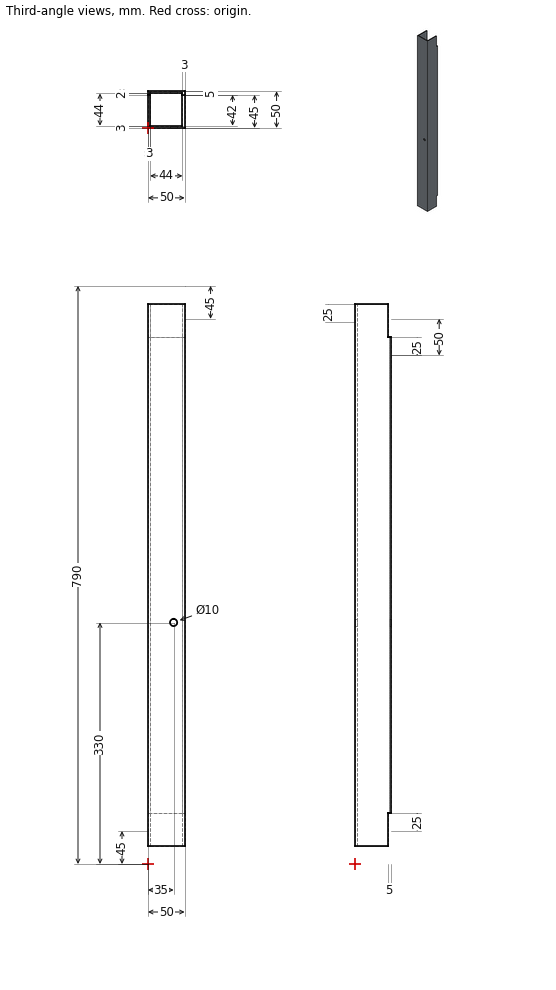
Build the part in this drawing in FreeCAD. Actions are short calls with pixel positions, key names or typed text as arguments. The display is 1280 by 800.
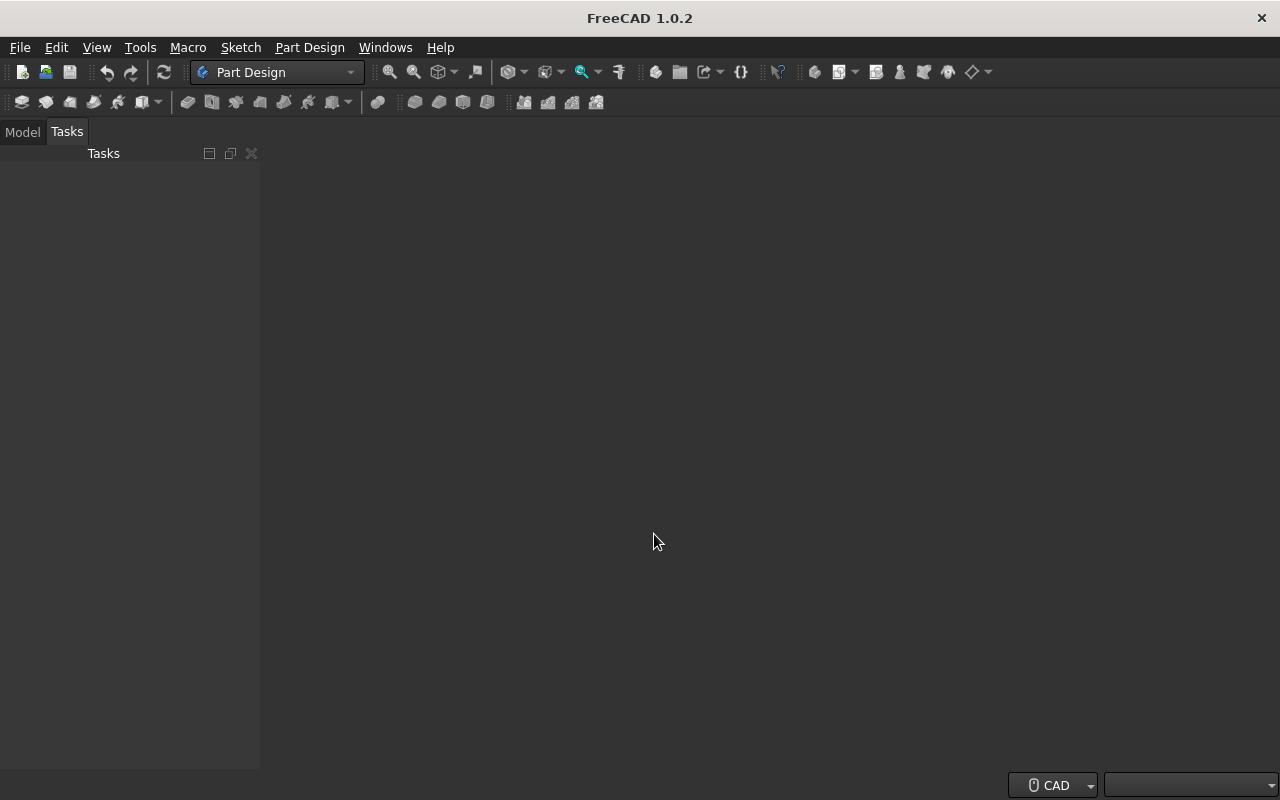
click(22, 72)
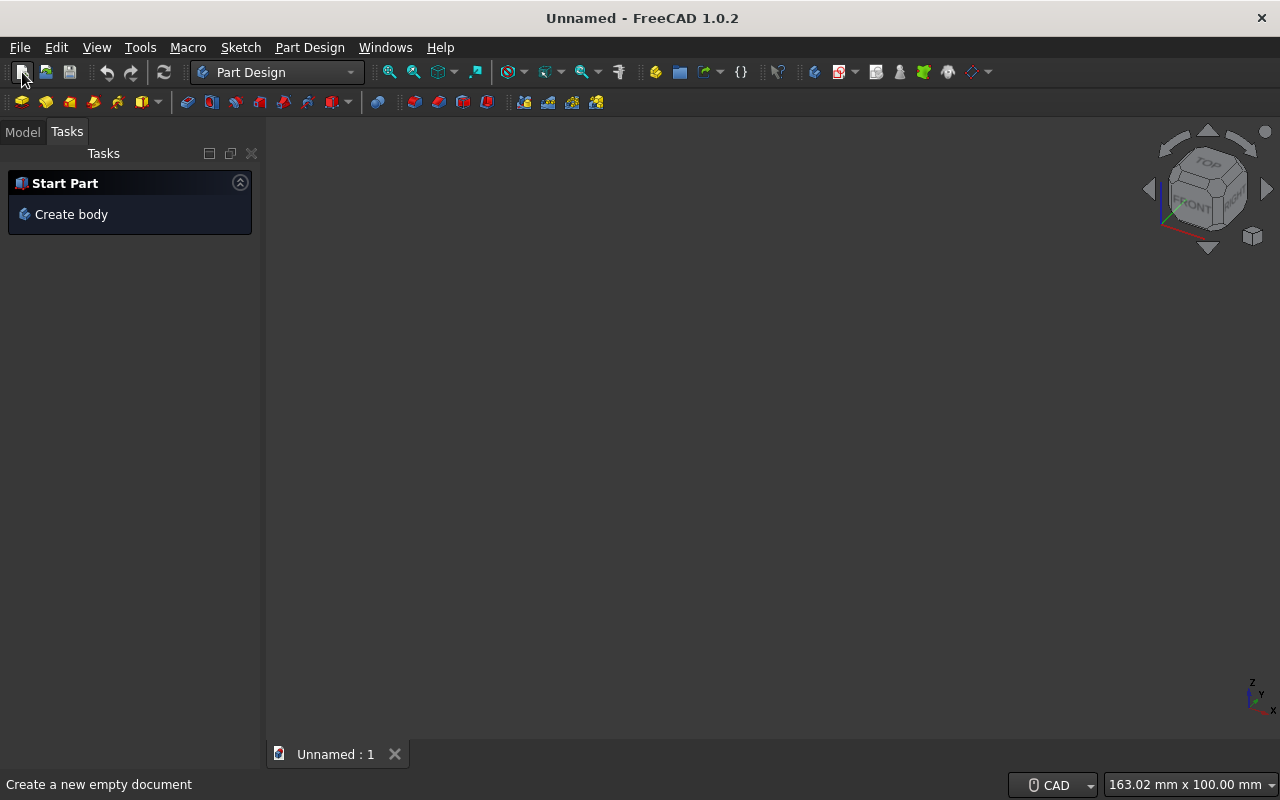
click(840, 72)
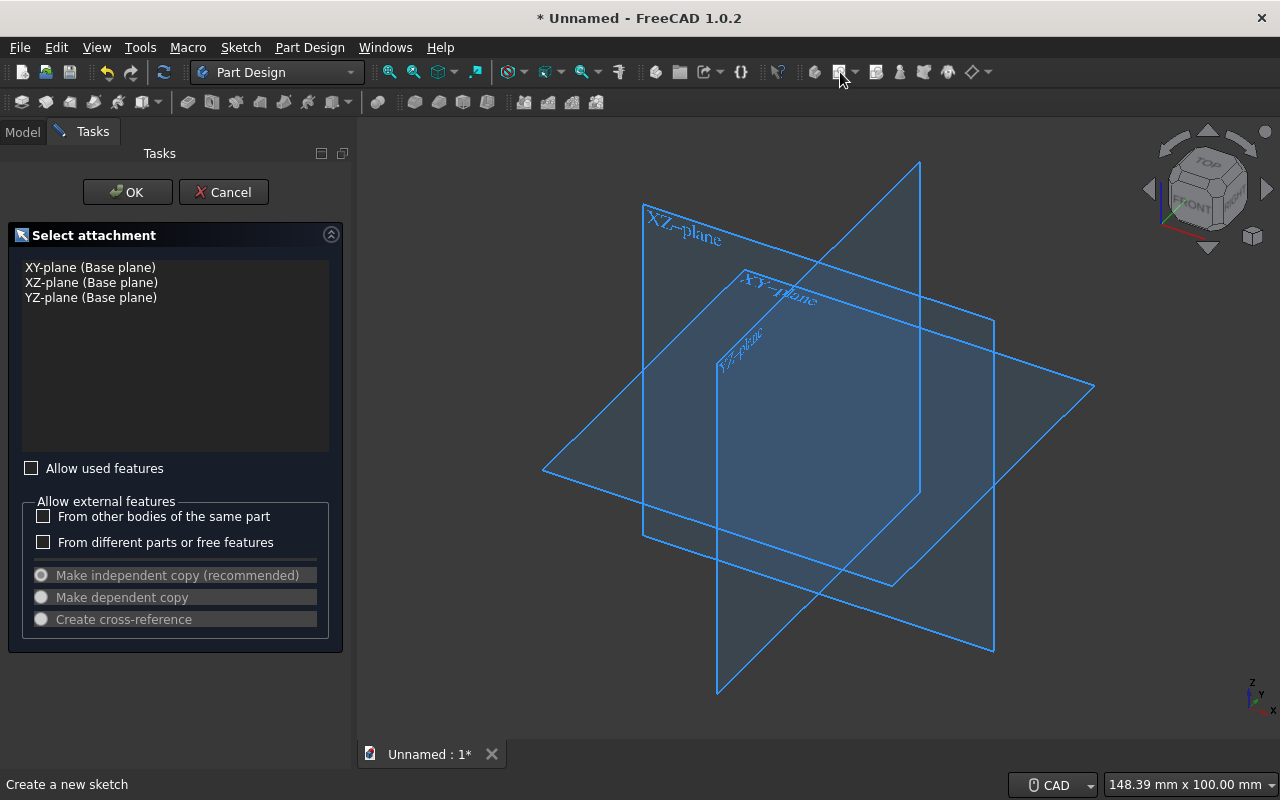
click(82, 268)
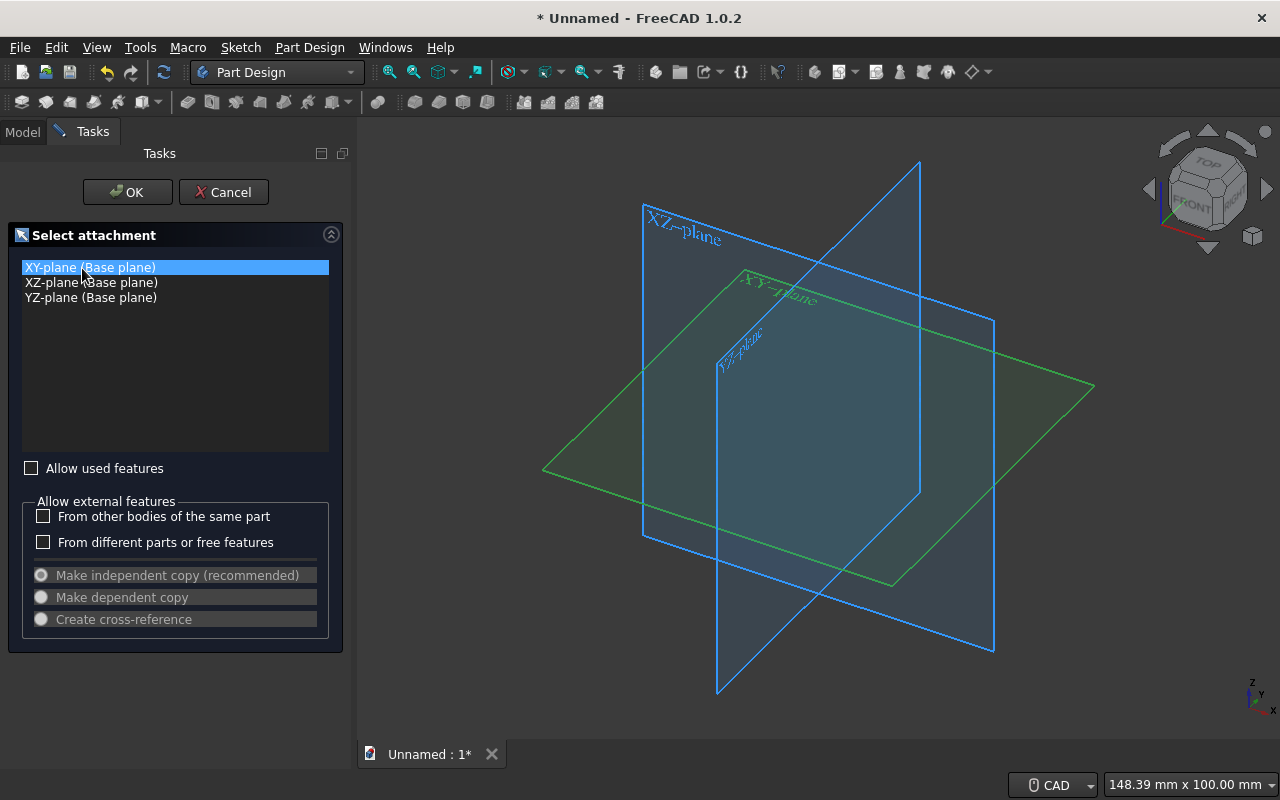
click(128, 192)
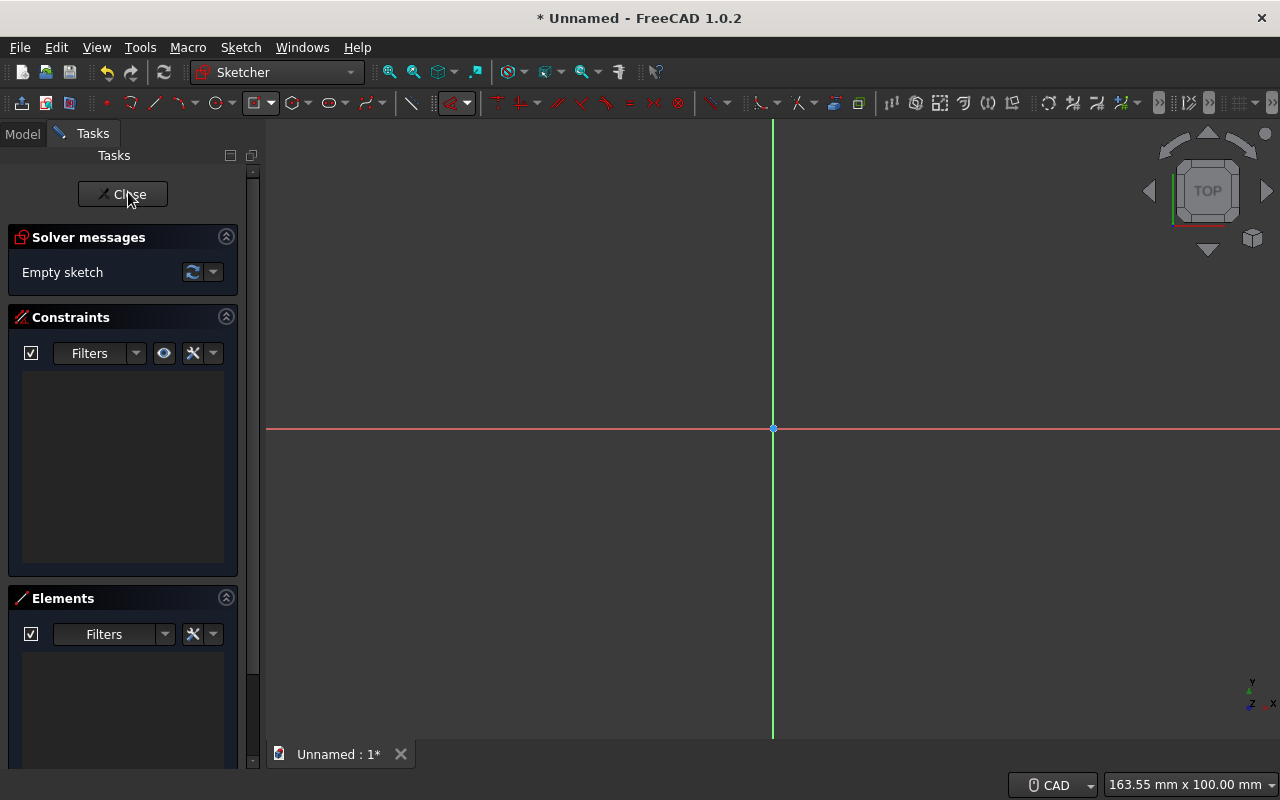
scroll(294, 711, down, 1)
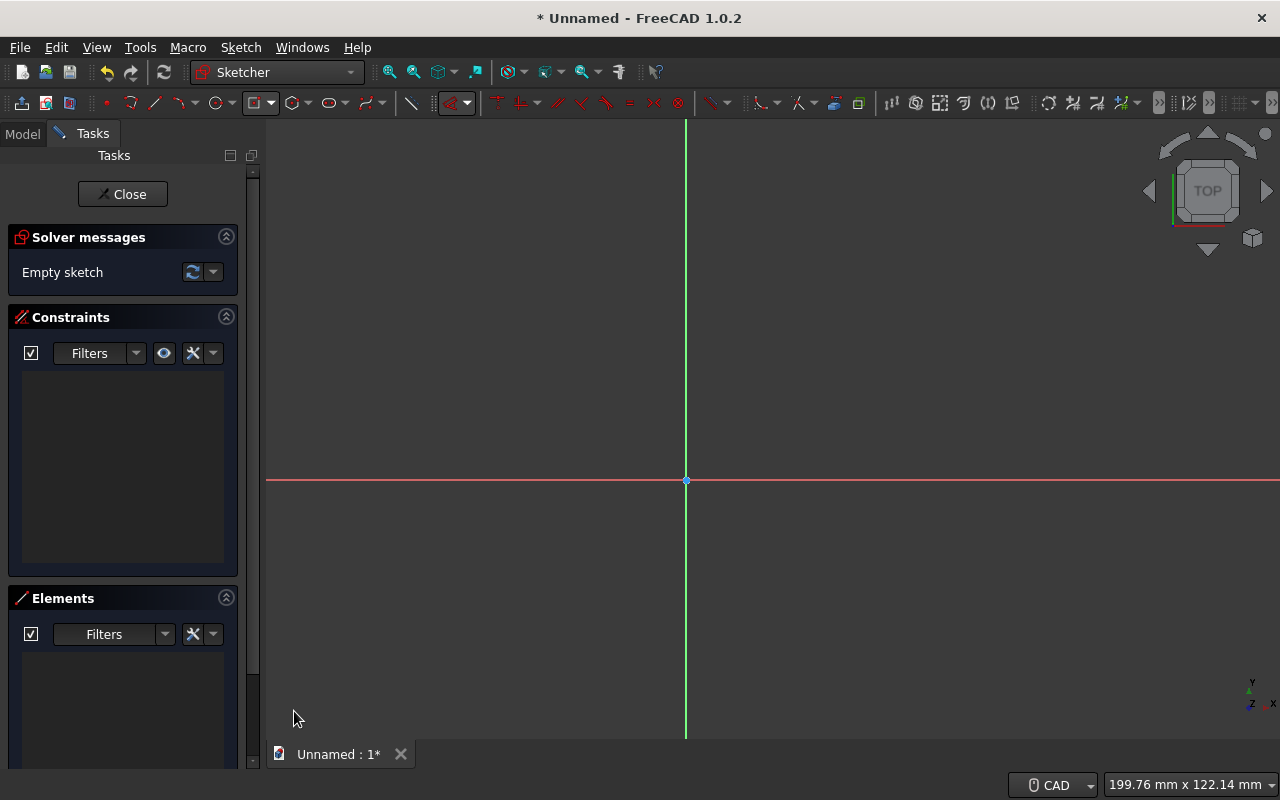
scroll(1034, 200, up, 2)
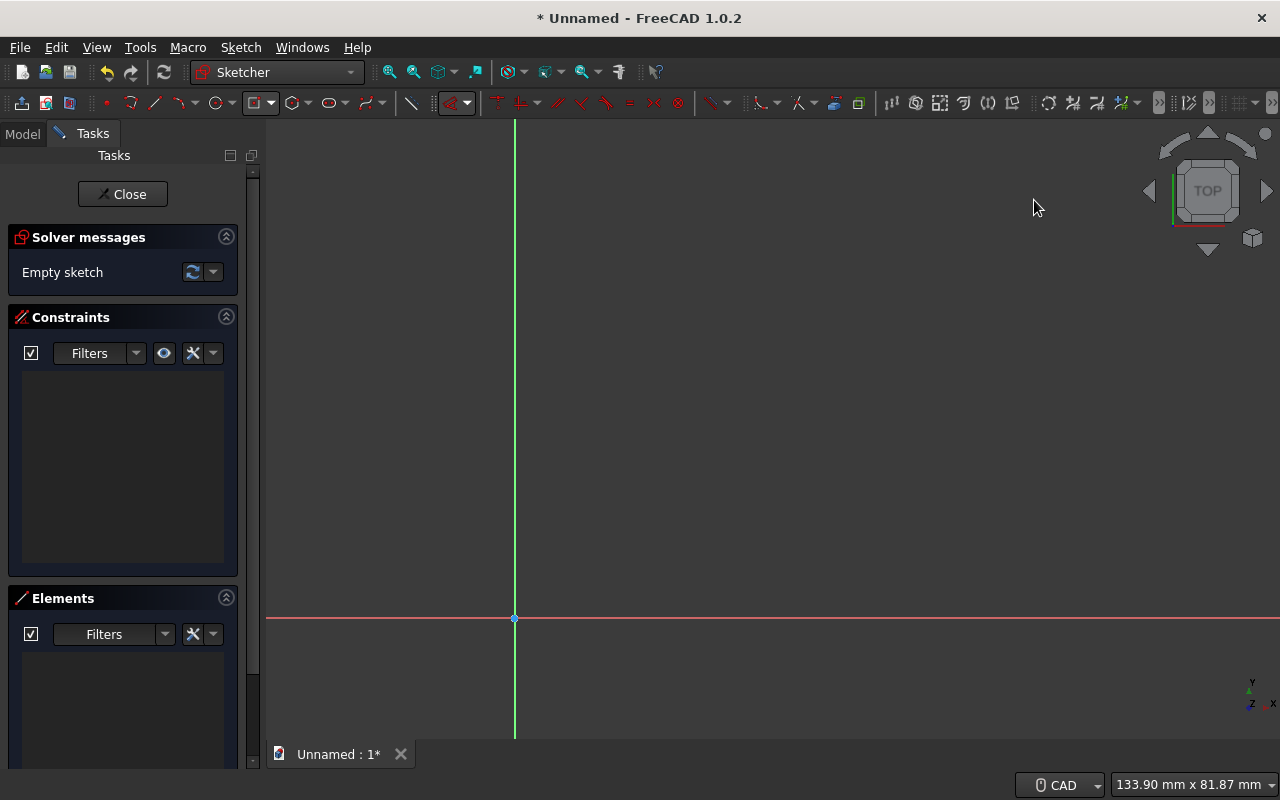
click(274, 104)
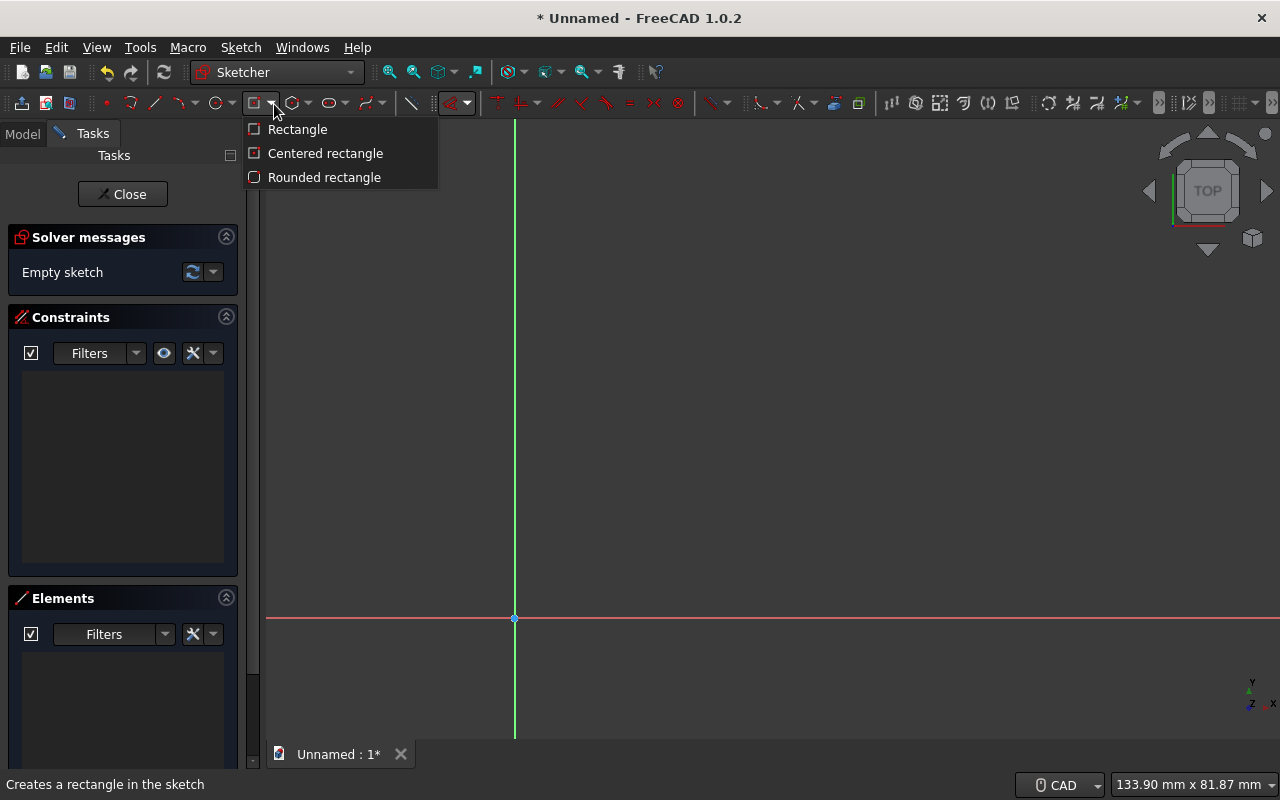
click(340, 129)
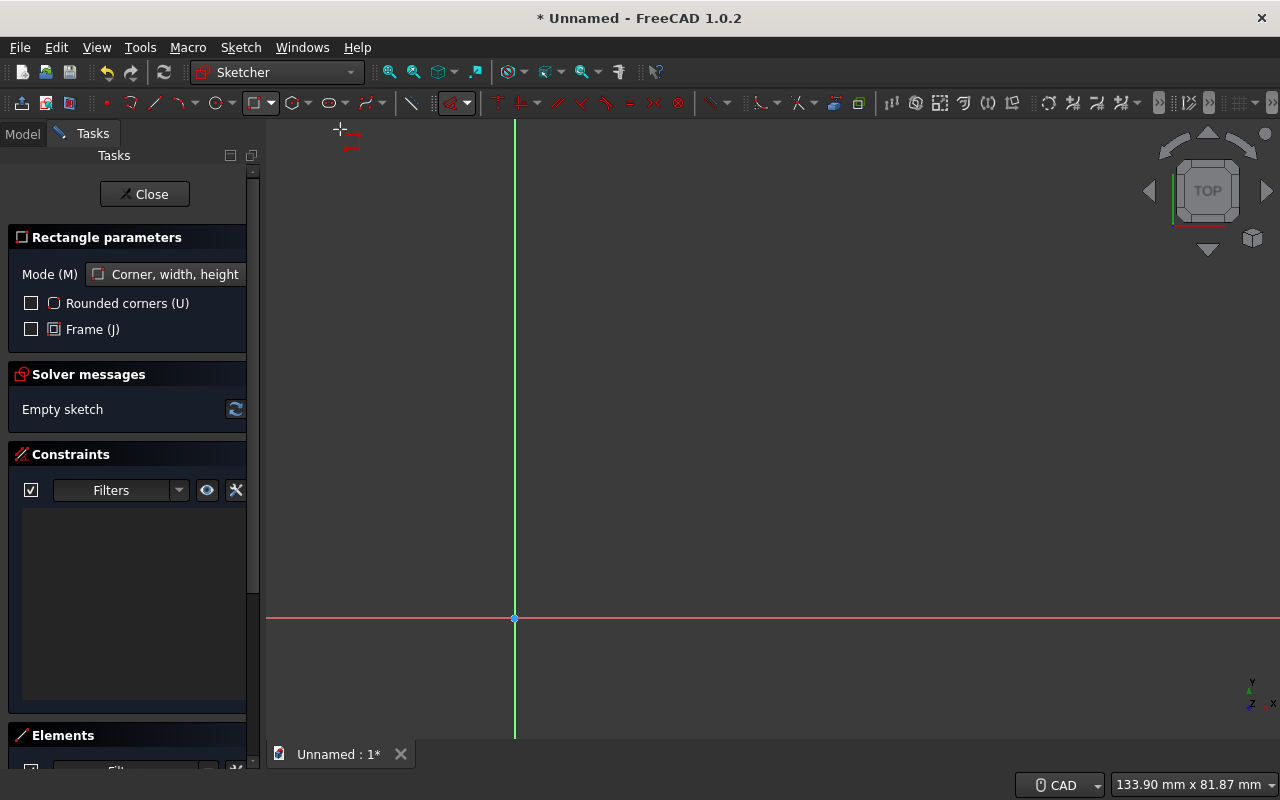
click(515, 618)
click(893, 239)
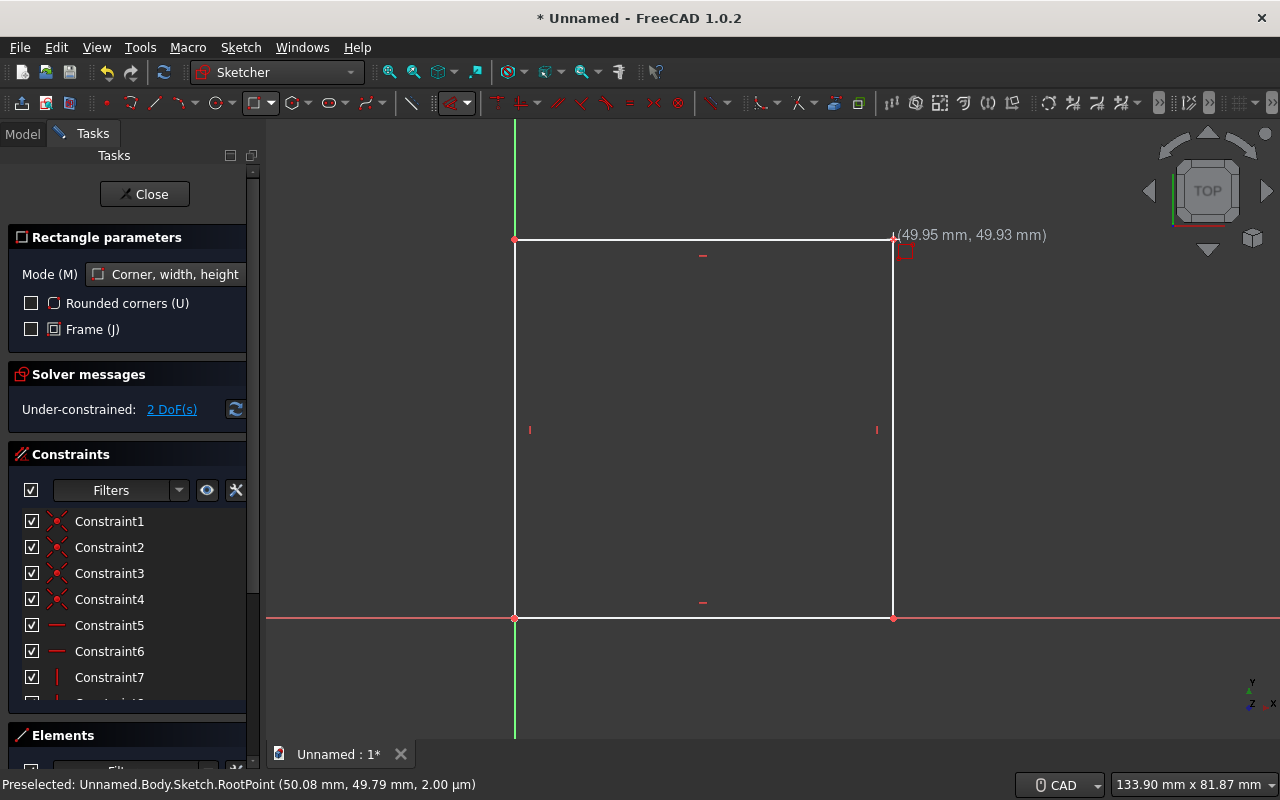
click(537, 262)
click(871, 595)
key(Escape)